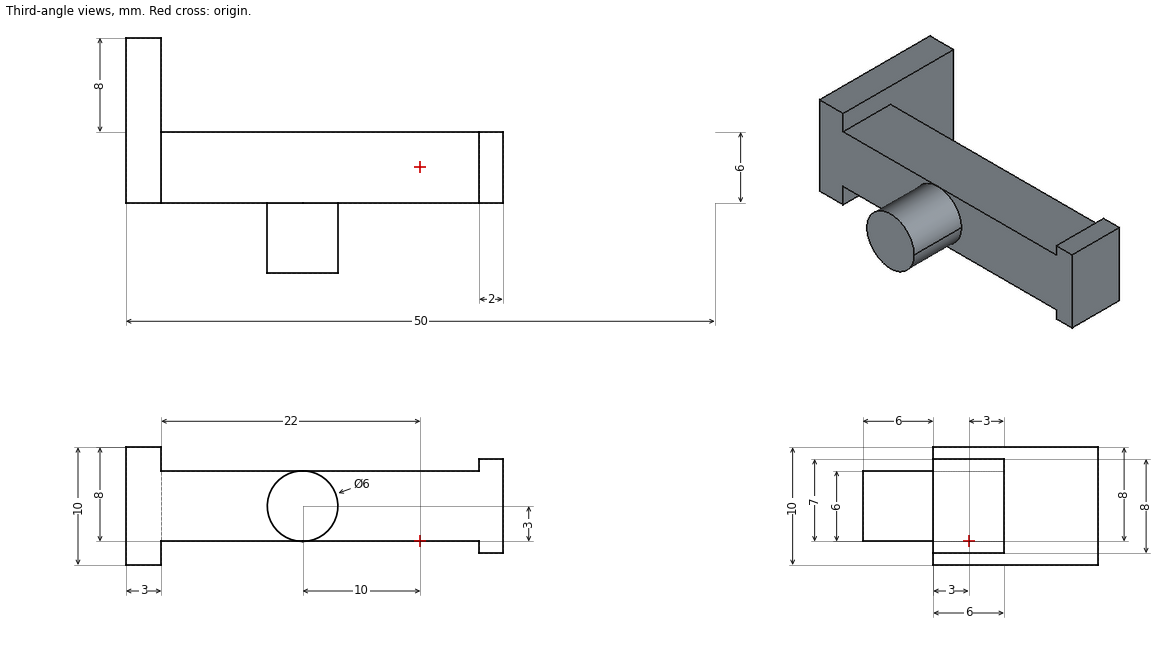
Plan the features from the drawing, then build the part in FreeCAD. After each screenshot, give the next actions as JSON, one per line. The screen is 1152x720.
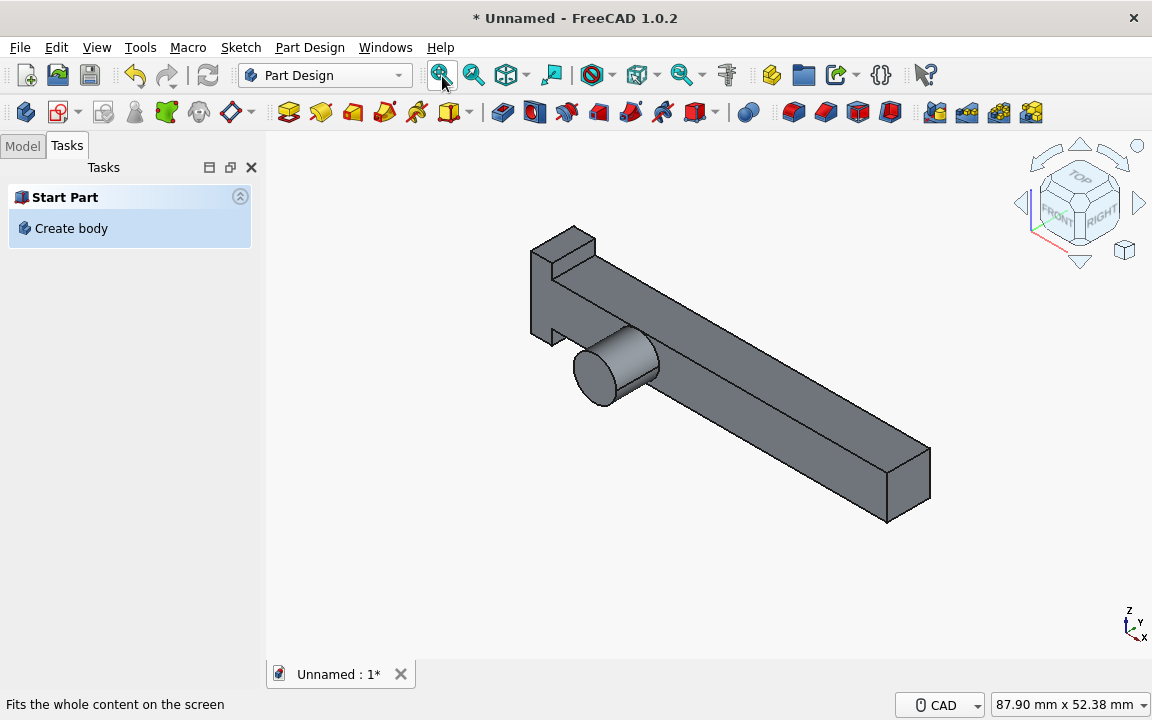
{"action": "left_click", "coordinate": [909, 485]}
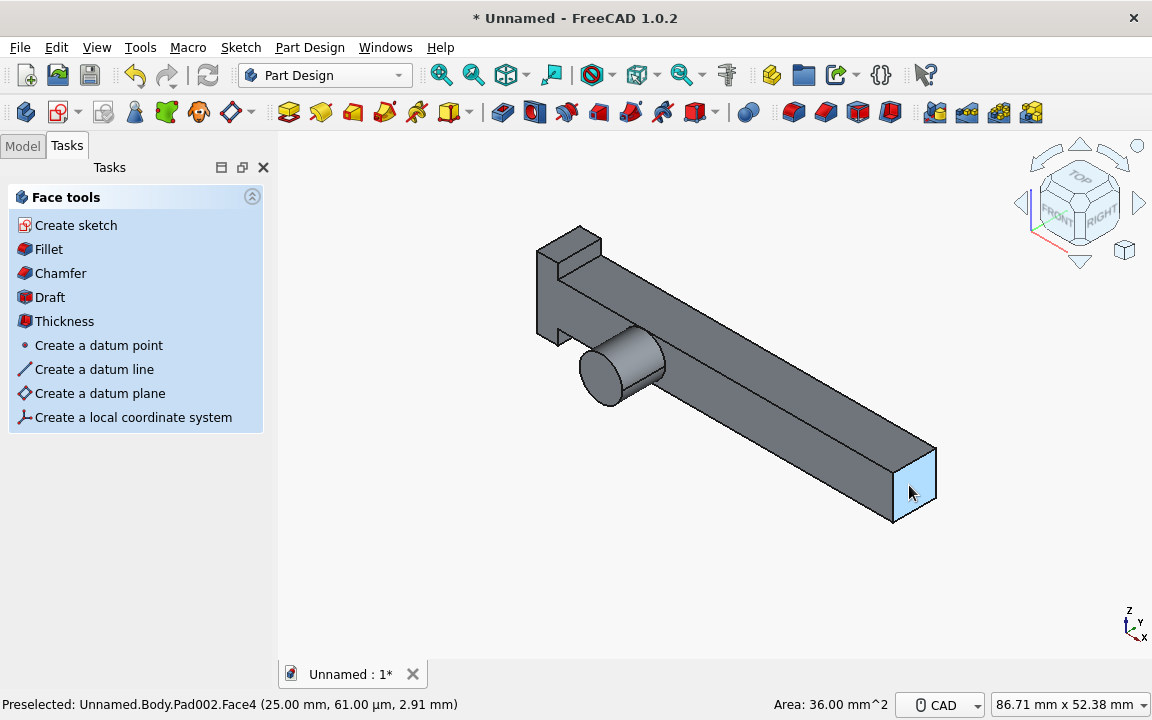
{"action": "left_click", "coordinate": [58, 112]}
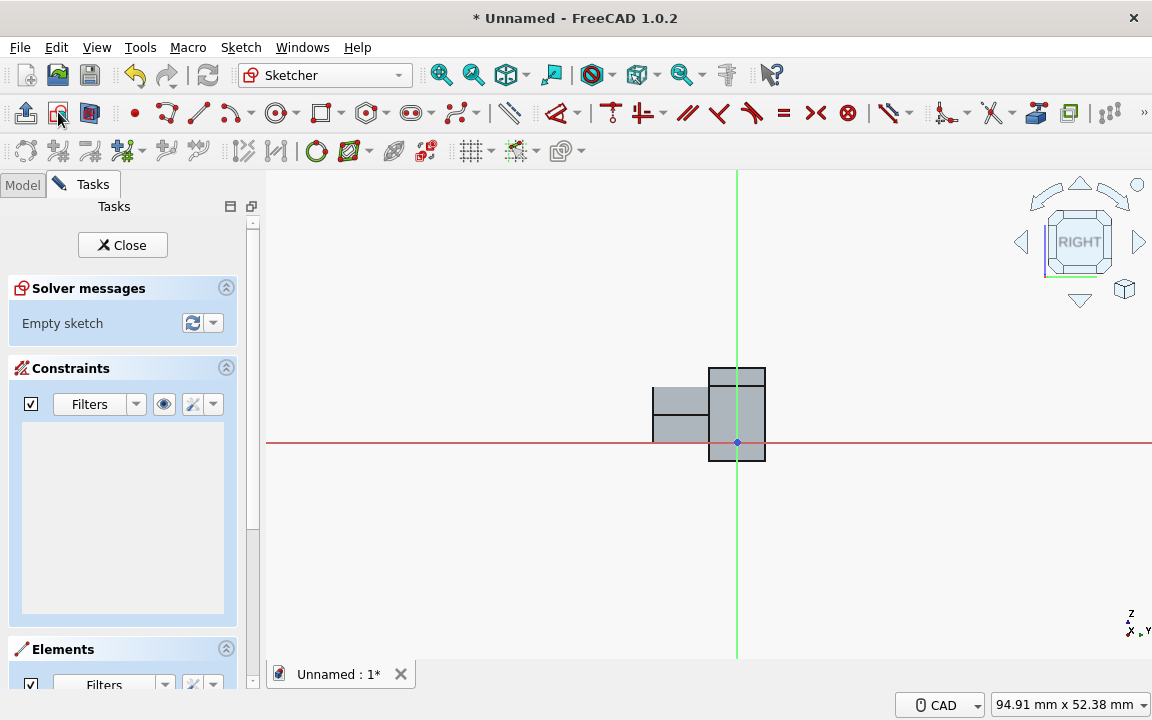
{"action": "scroll", "coordinate": [761, 414], "scroll_direction": "up", "scroll_amount": 8}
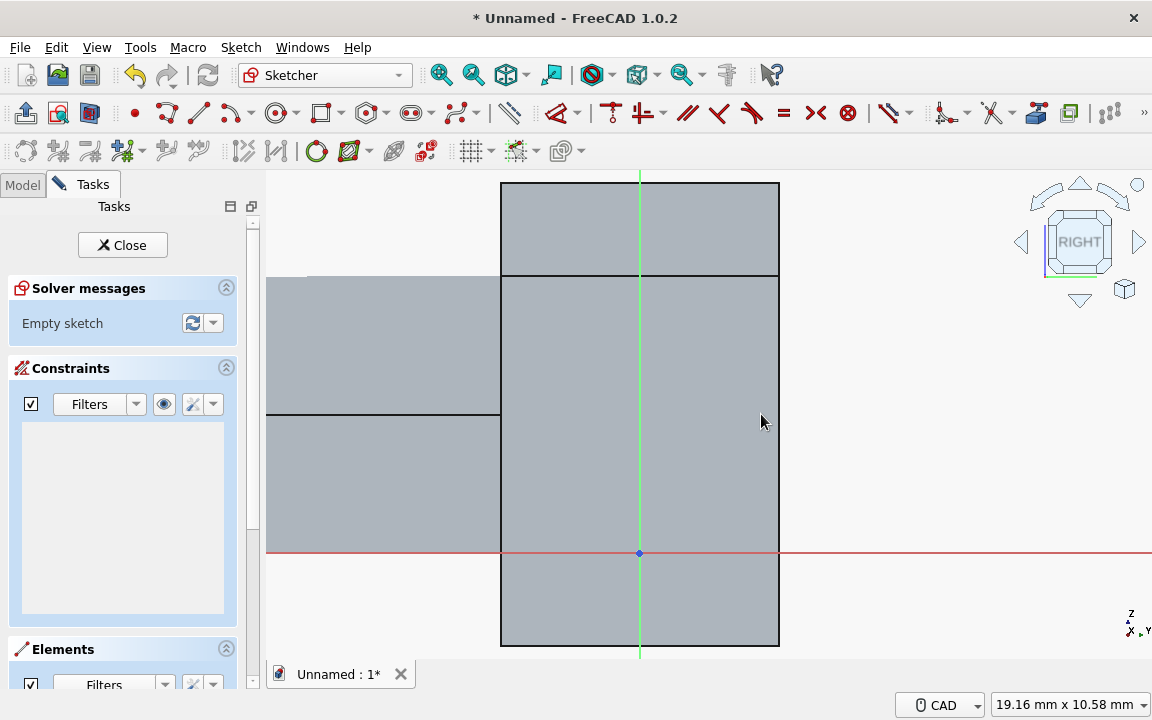
{"action": "left_click", "coordinate": [322, 114]}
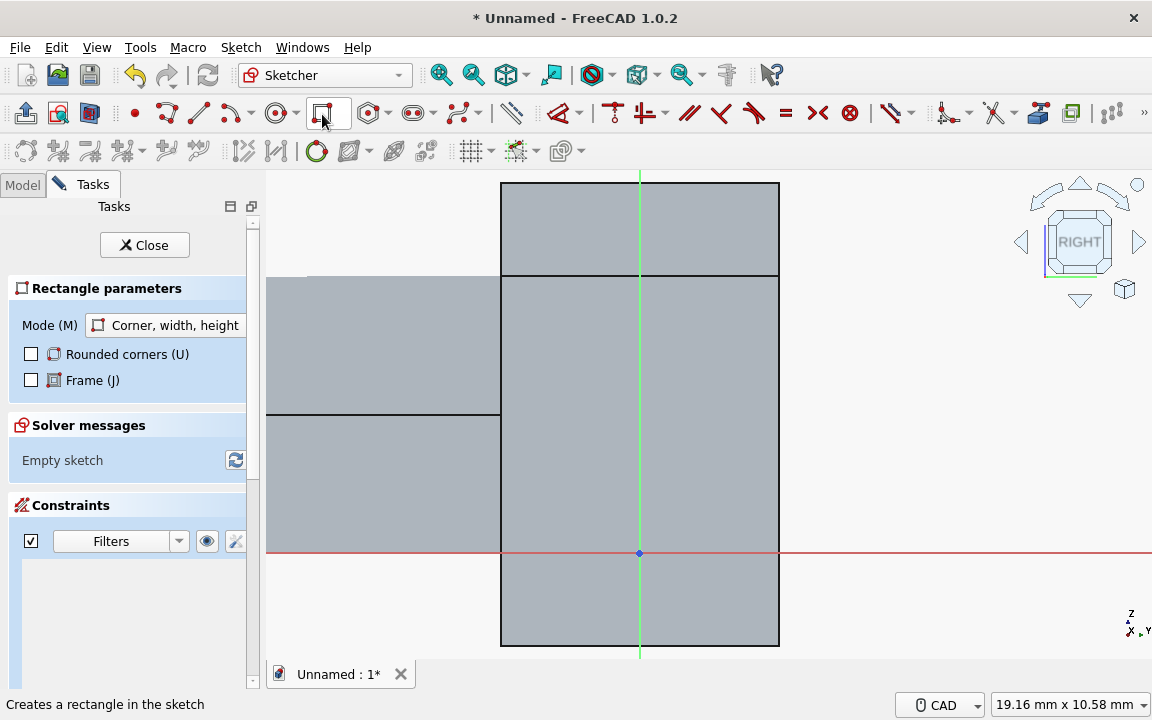
{"action": "left_click", "coordinate": [501, 276]}
{"action": "left_click", "coordinate": [779, 553]}
{"action": "key", "text": "Escape"}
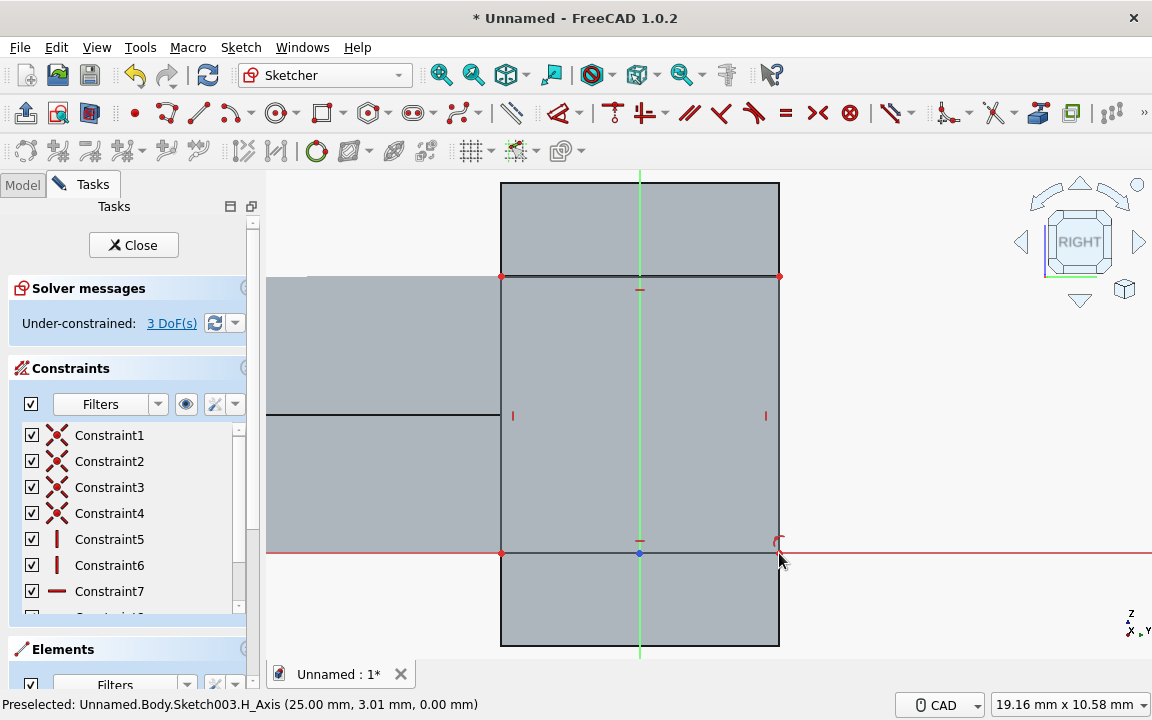
{"action": "left_click", "coordinate": [558, 114]}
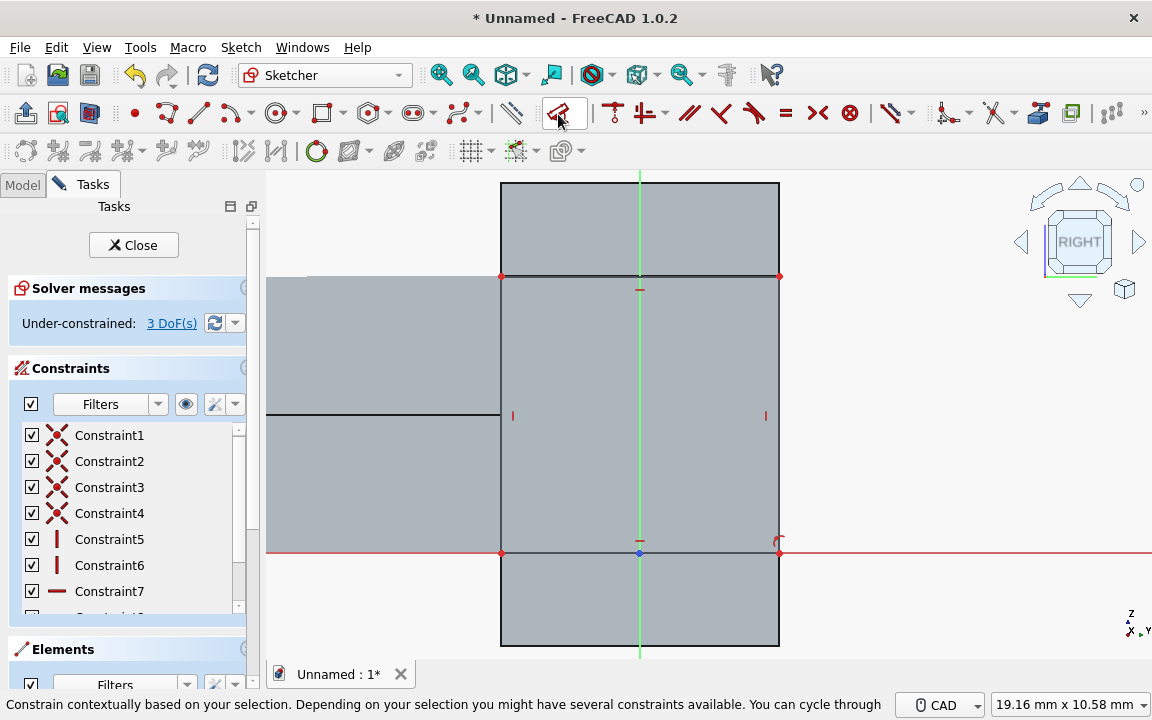
{"action": "left_click", "coordinate": [501, 360]}
{"action": "left_click", "coordinate": [467, 415]}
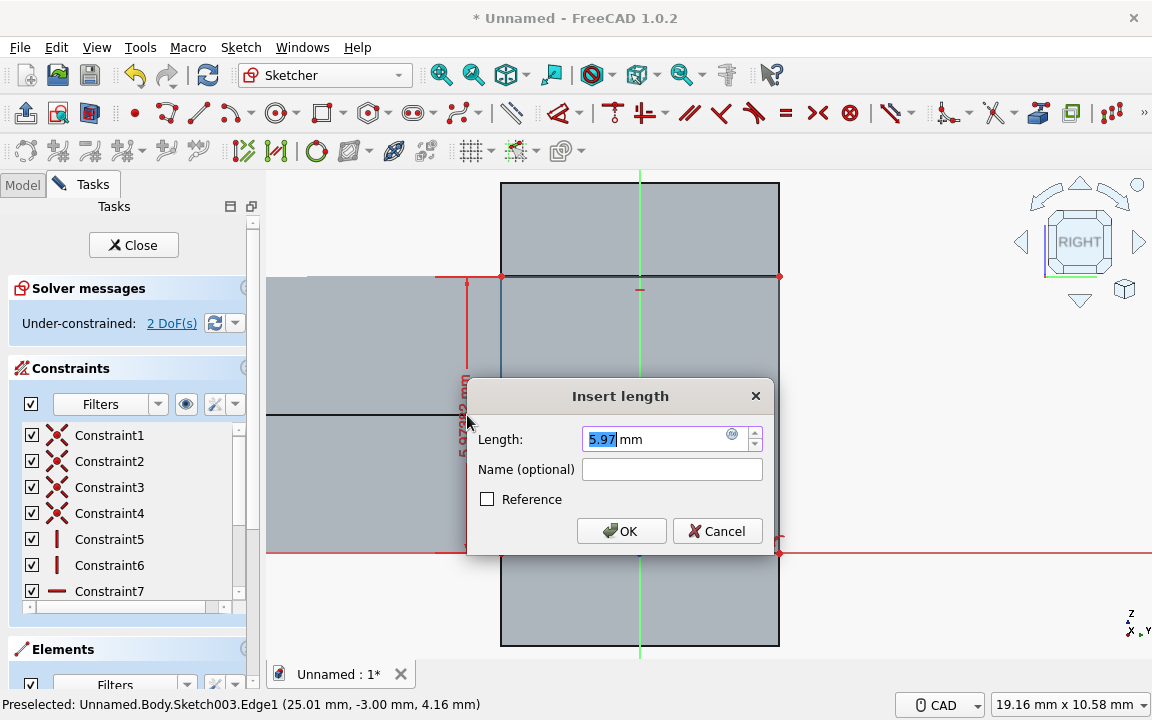
{"action": "type", "text": "6"}
{"action": "key", "text": "Return"}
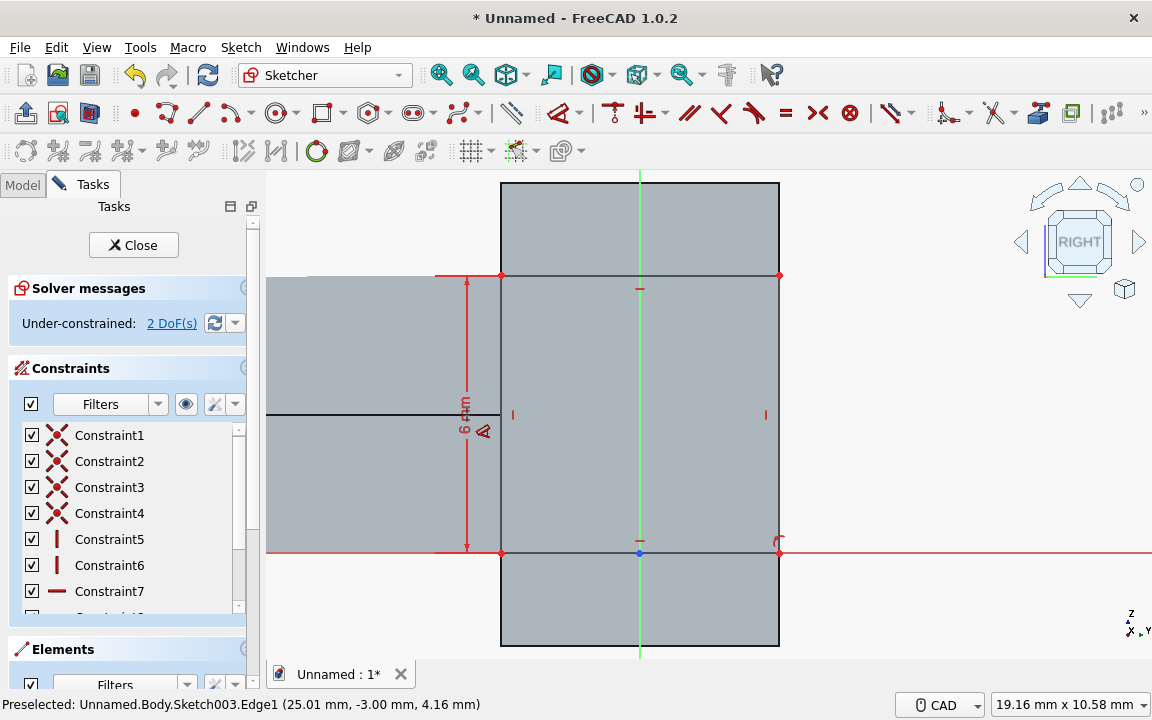
{"action": "left_click", "coordinate": [584, 553]}
{"action": "left_click", "coordinate": [576, 587]}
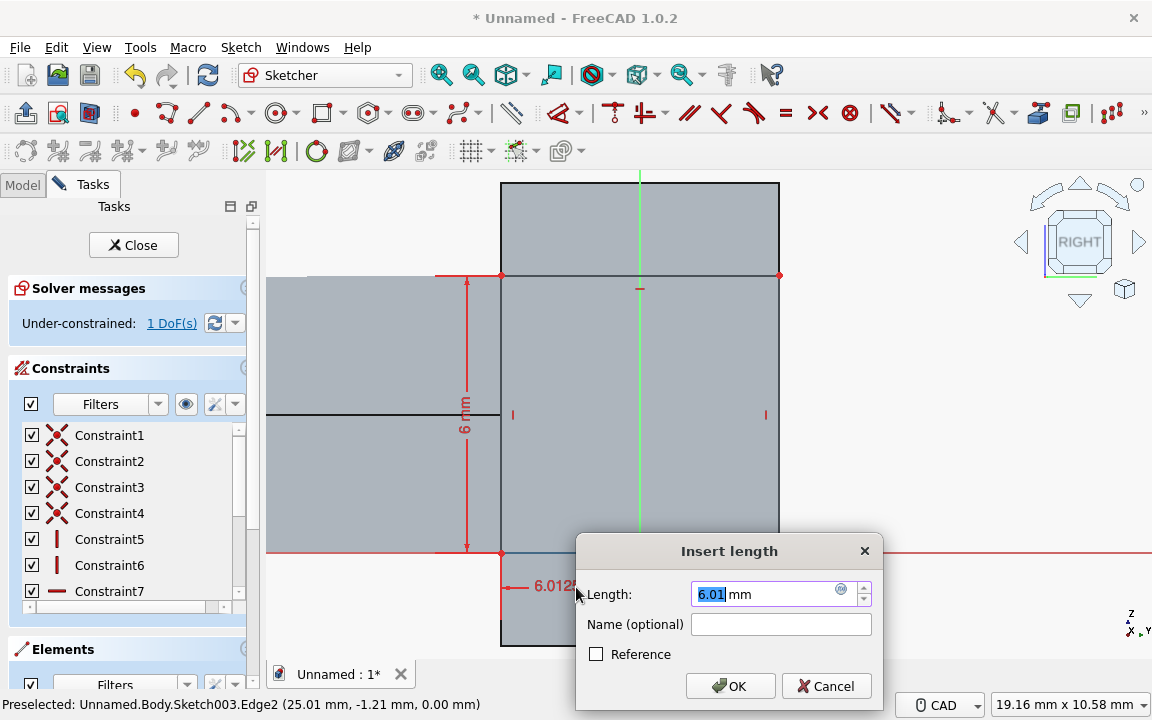
{"action": "type", "text": "6"}
{"action": "key", "text": "Return"}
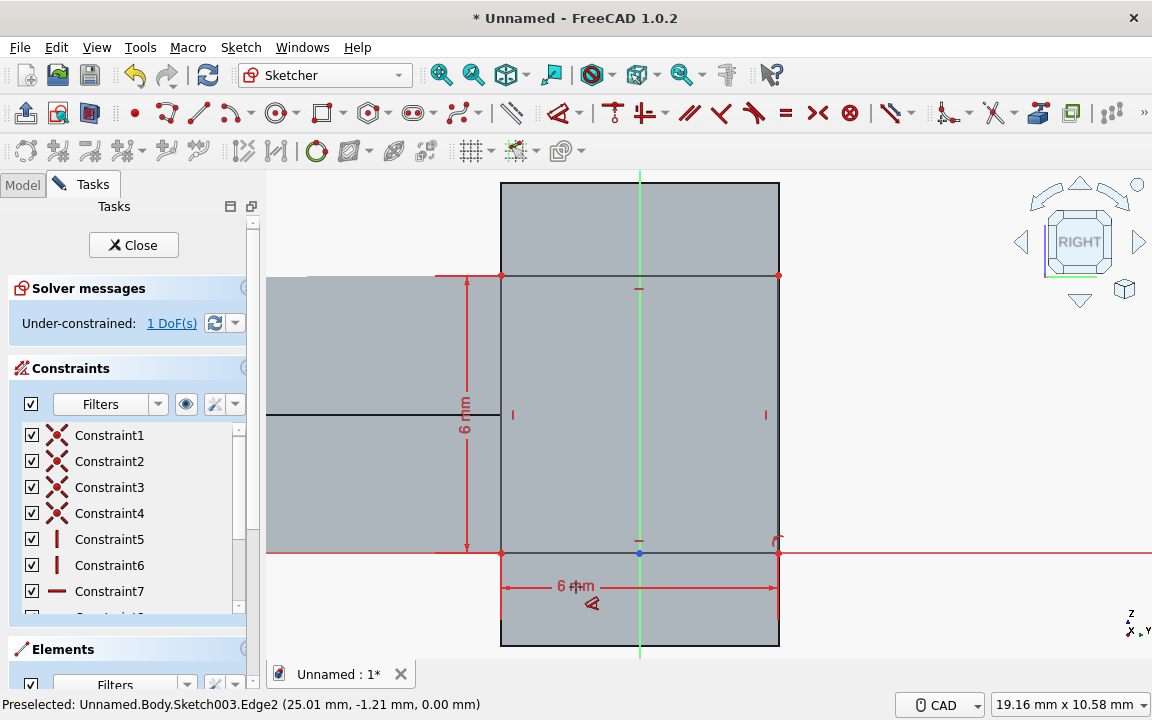
{"action": "left_click", "coordinate": [501, 276]}
{"action": "left_click", "coordinate": [570, 242]}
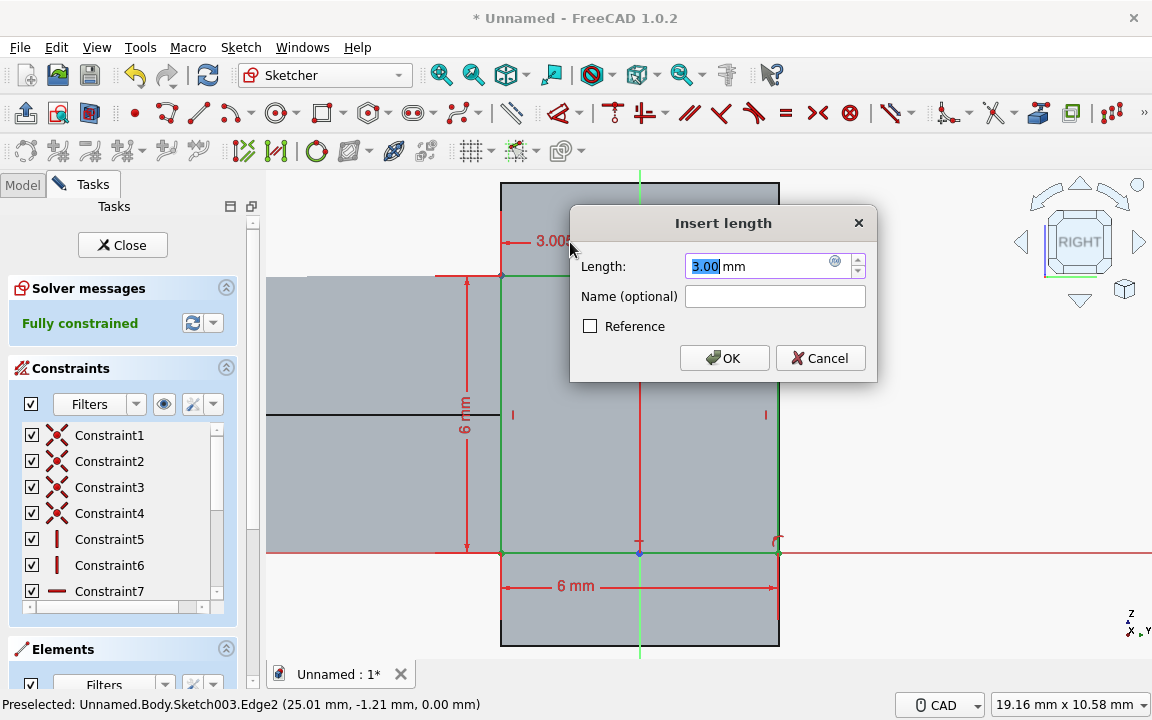
{"action": "type", "text": "3"}
{"action": "key", "text": "Return"}
{"action": "key", "text": "Escape"}